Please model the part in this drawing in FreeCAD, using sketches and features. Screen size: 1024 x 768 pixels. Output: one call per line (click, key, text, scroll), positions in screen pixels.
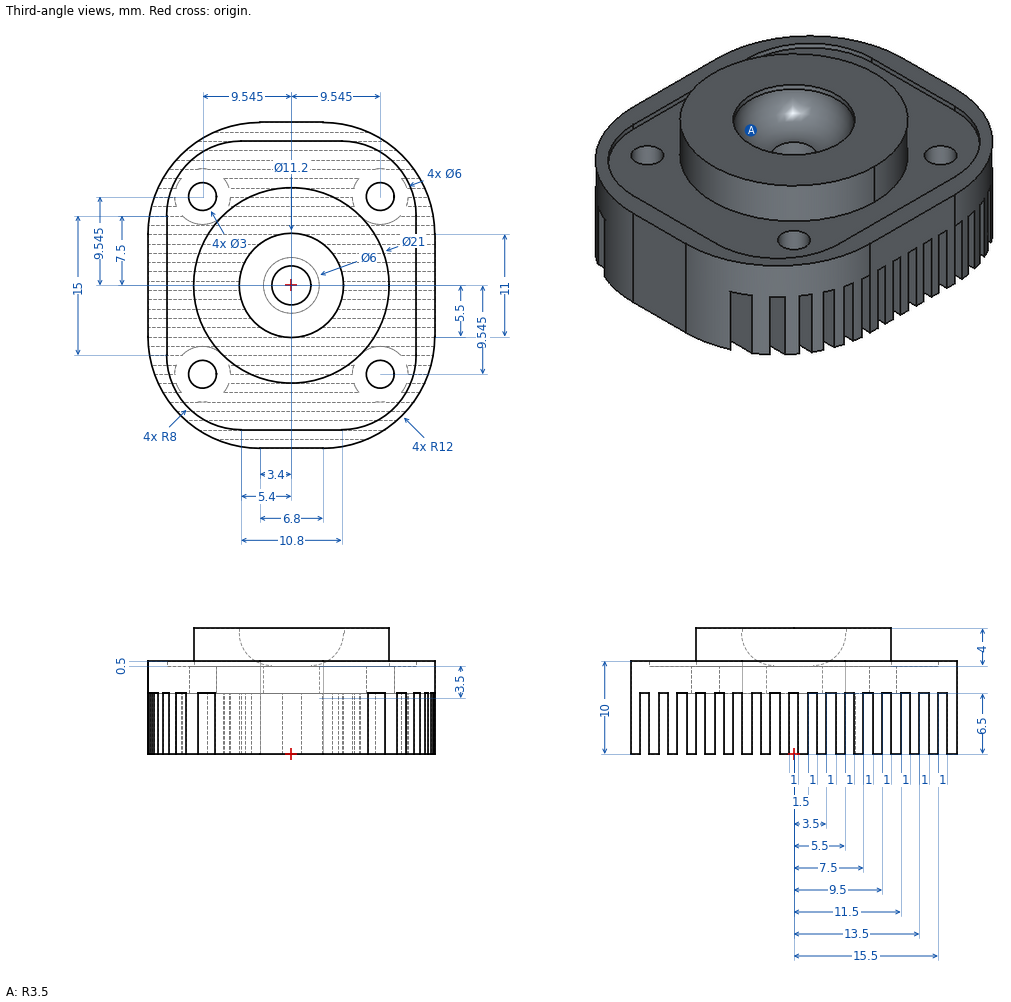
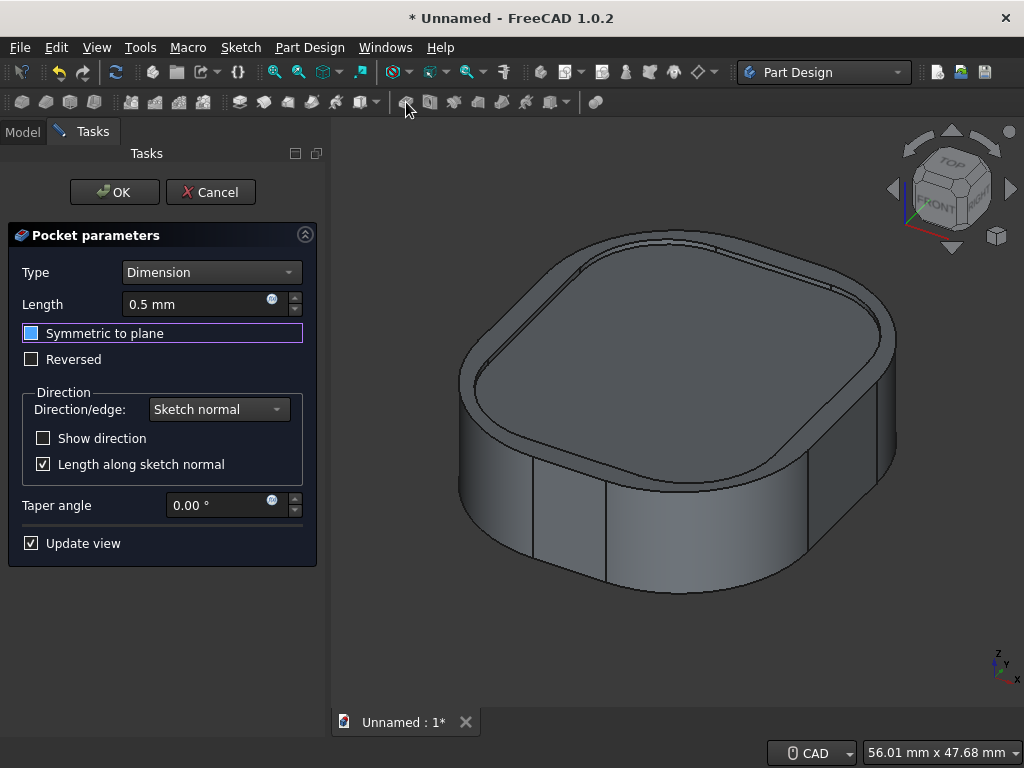
click(115, 192)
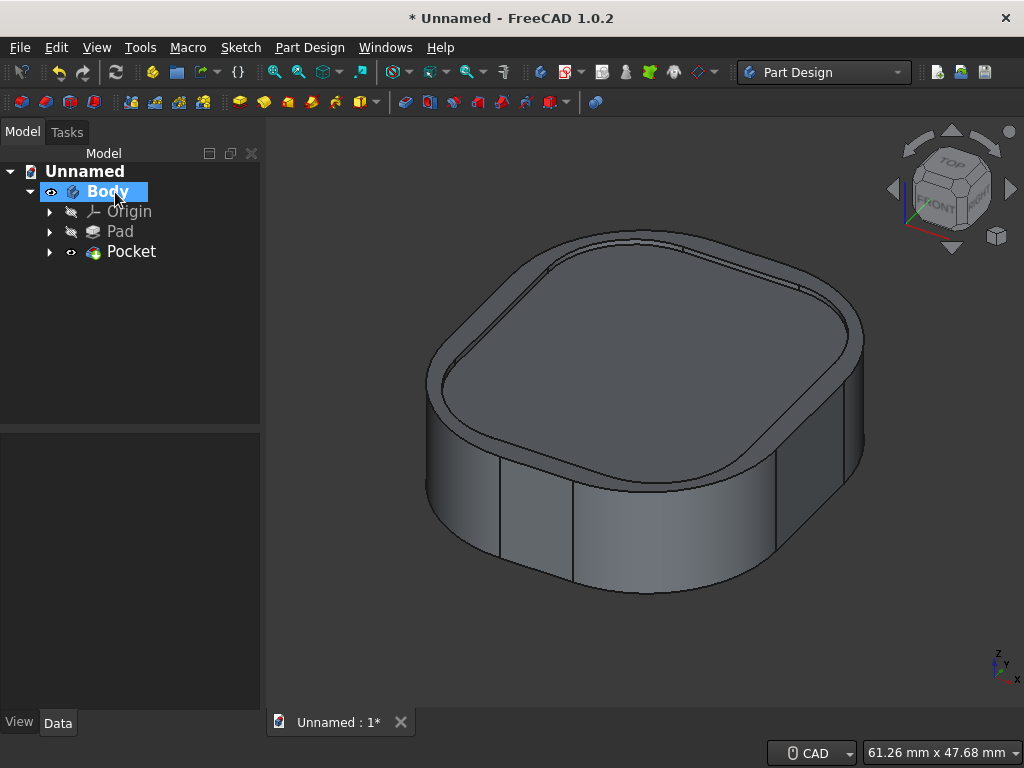
click(645, 365)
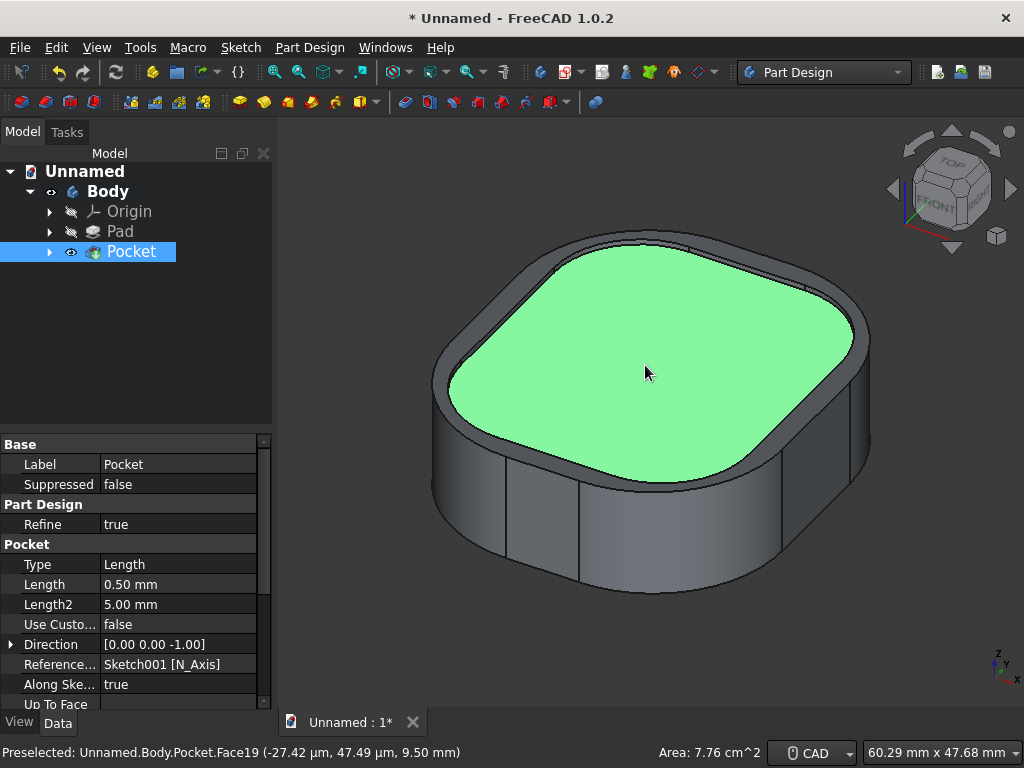
click(566, 72)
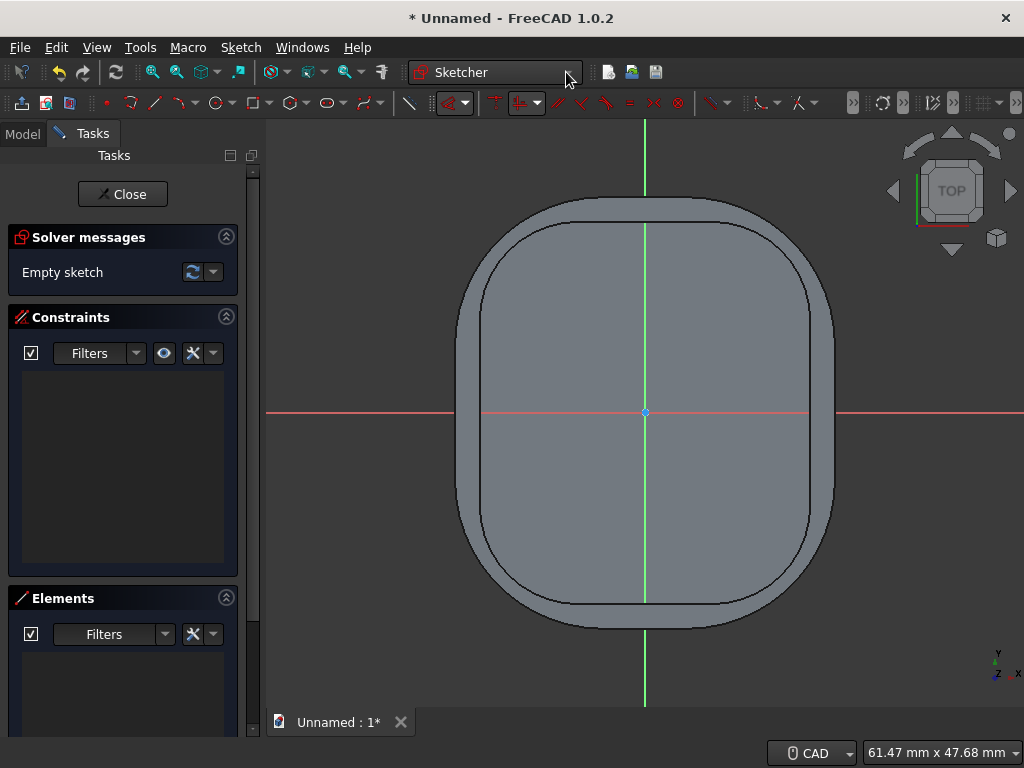
scroll(784, 413, up, 2)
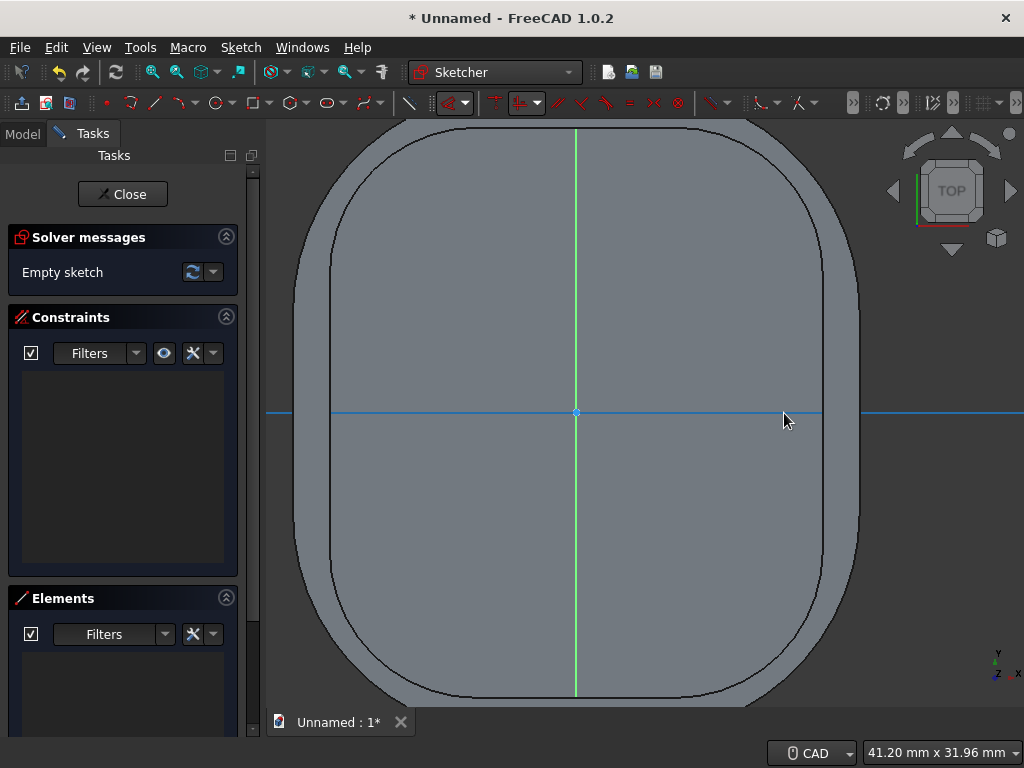
click(216, 104)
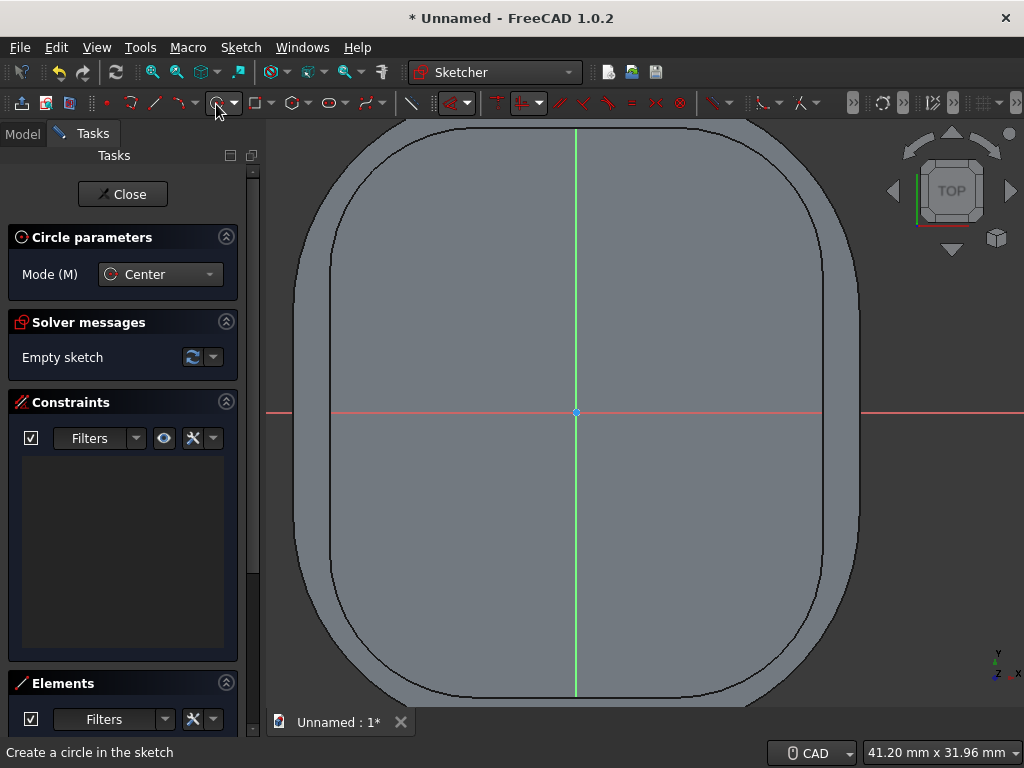
click(576, 413)
move(713, 276)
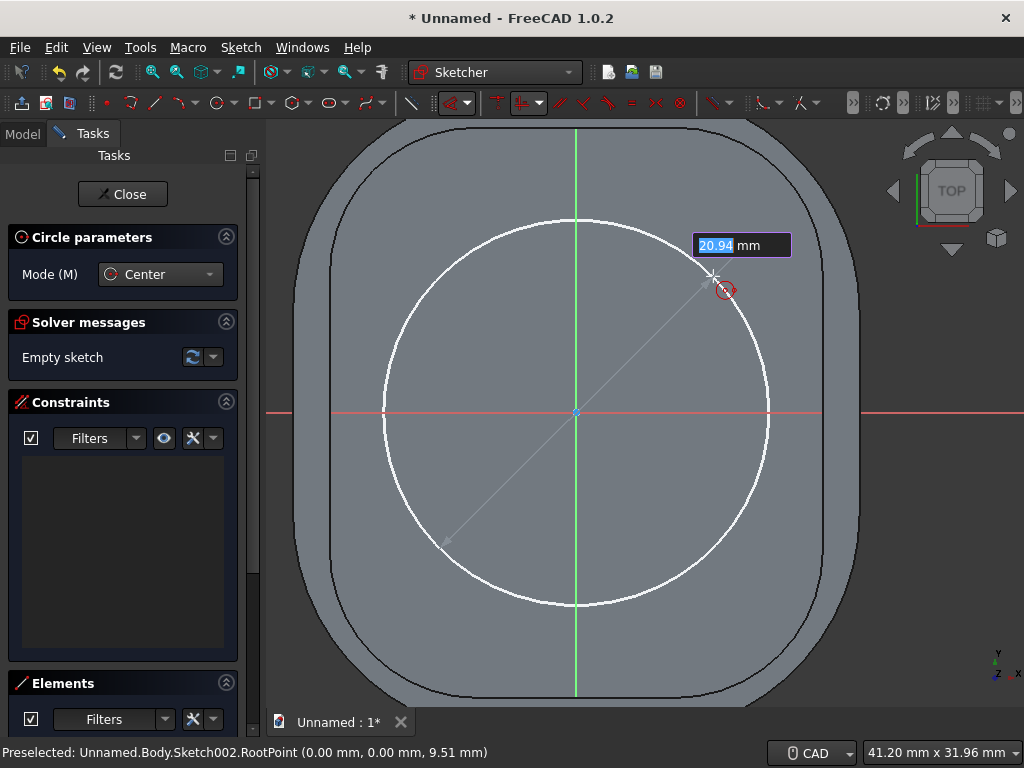
text(21)
key(Return)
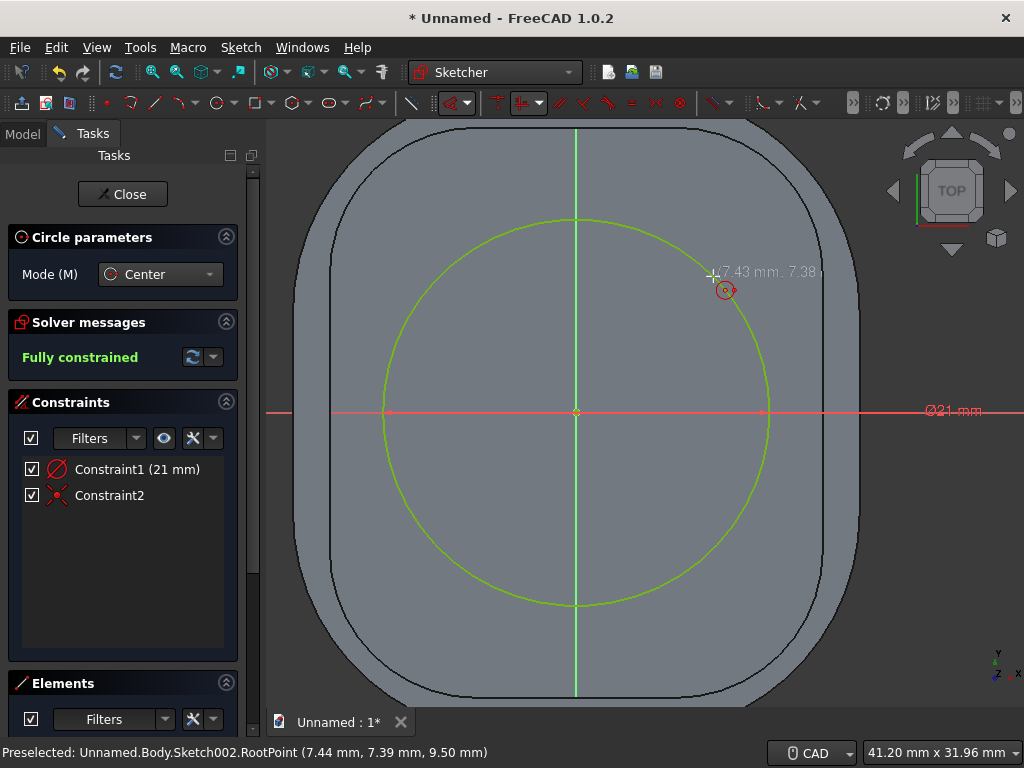
click(576, 413)
move(649, 340)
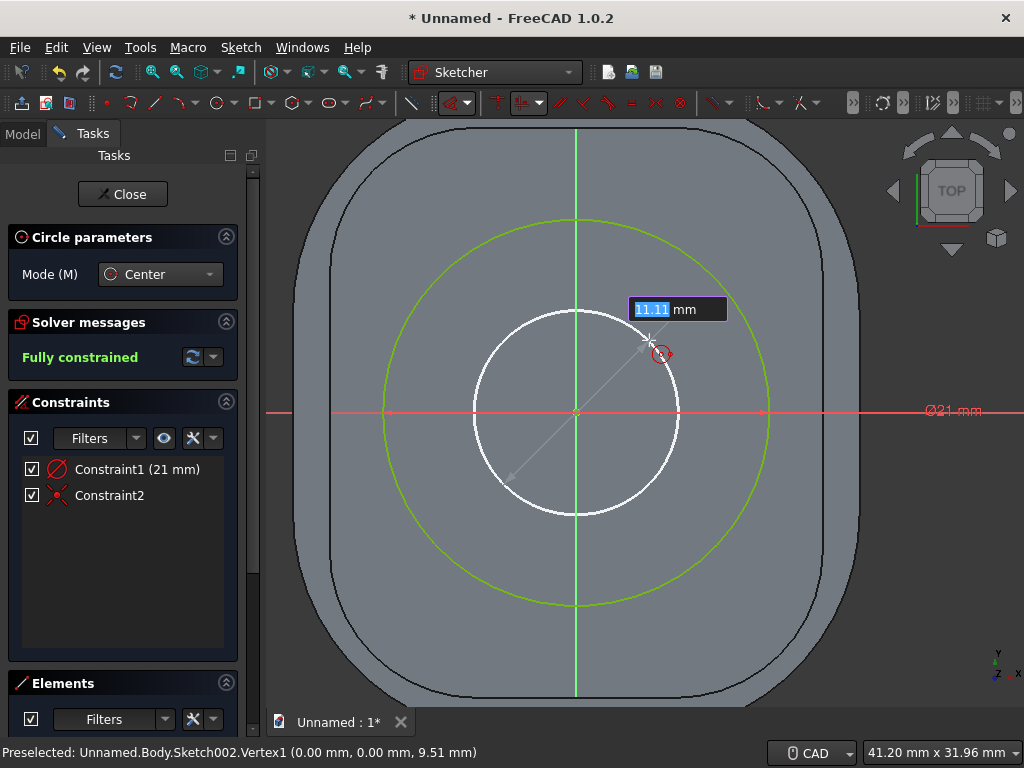
text(11.2)
key(Return)
key(Escape)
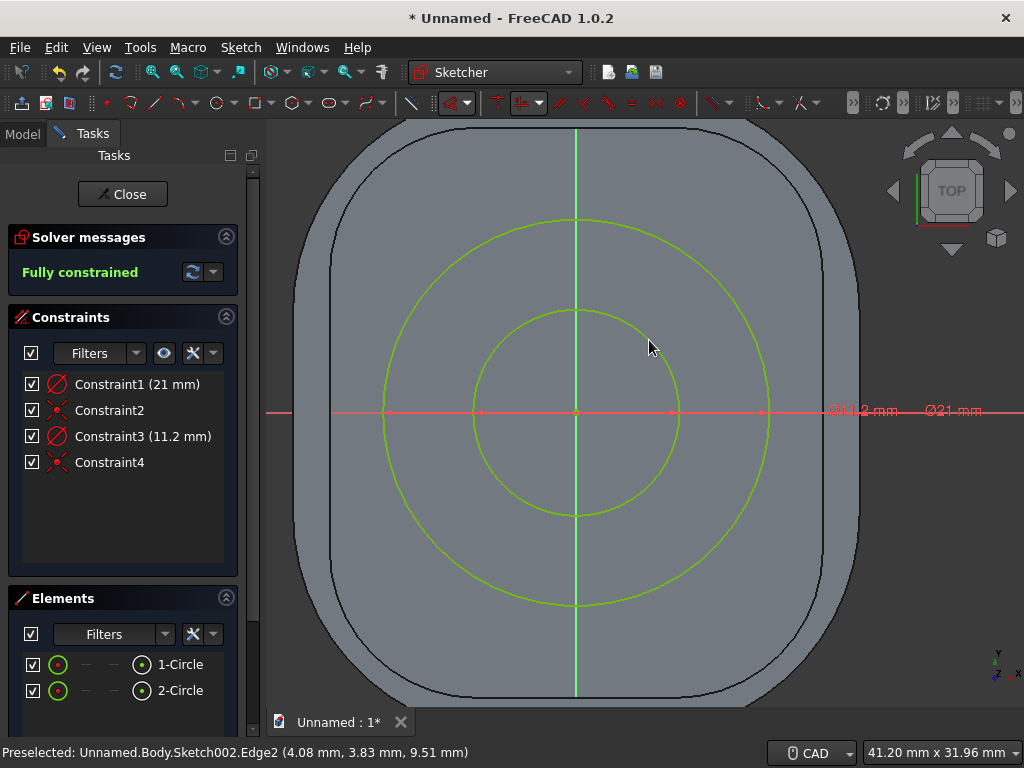
click(123, 194)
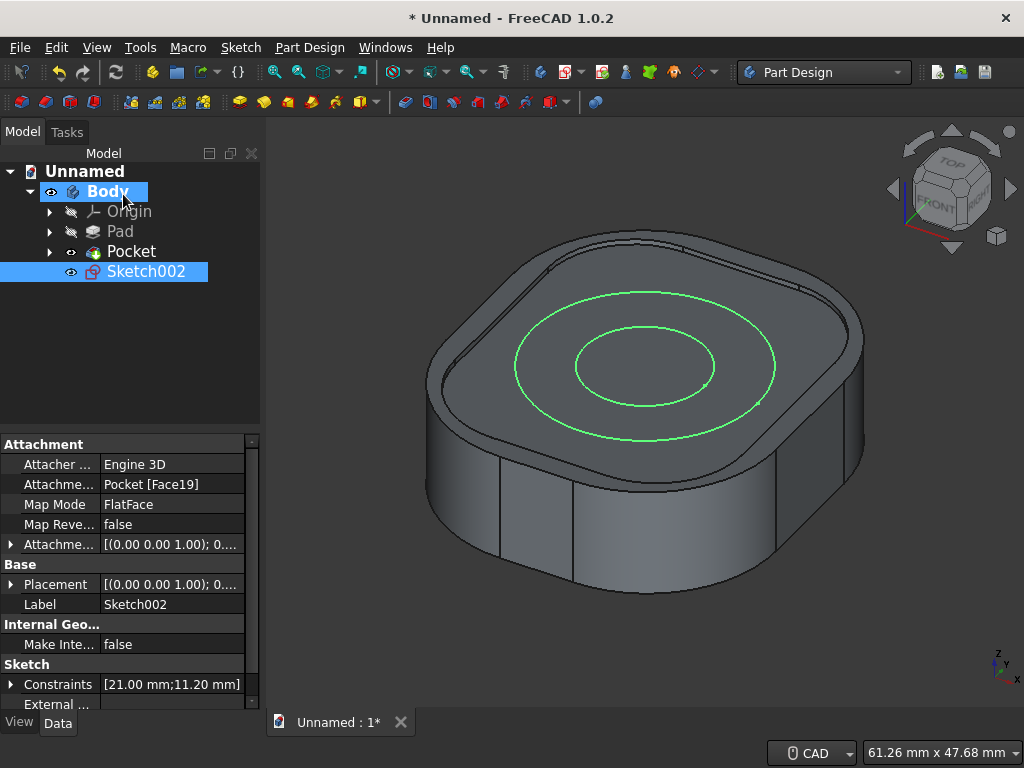
click(240, 102)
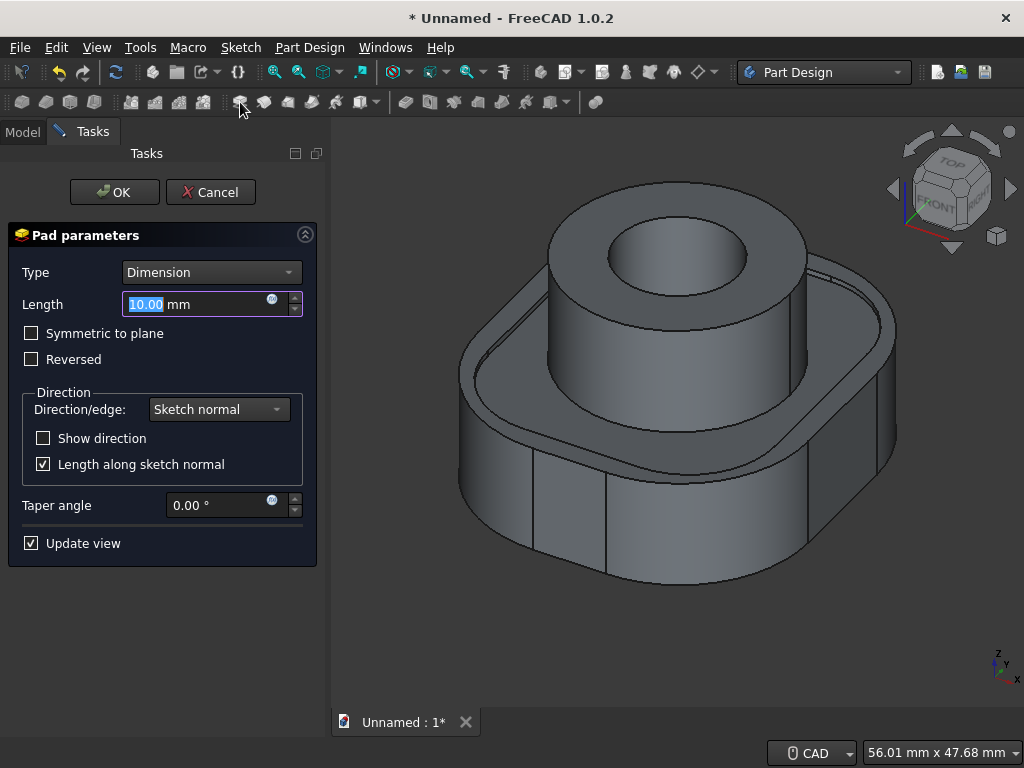
text(4)
key(Tab)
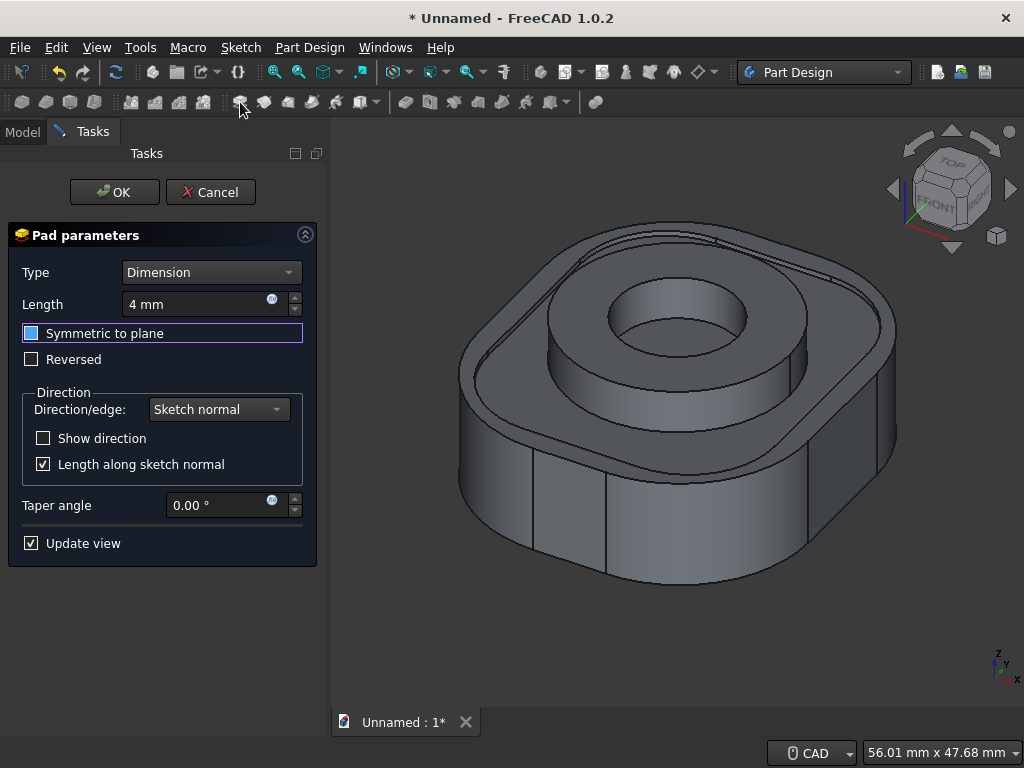
click(115, 192)